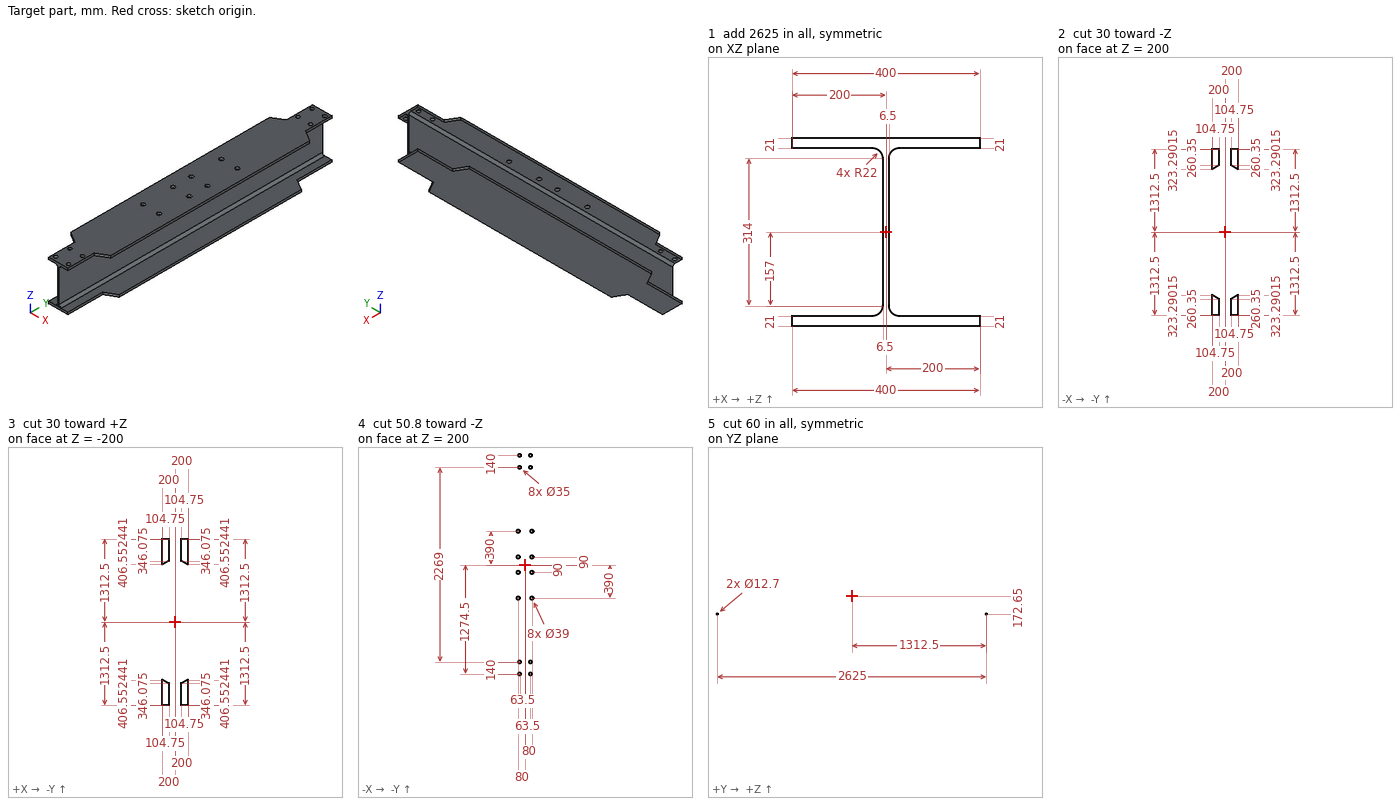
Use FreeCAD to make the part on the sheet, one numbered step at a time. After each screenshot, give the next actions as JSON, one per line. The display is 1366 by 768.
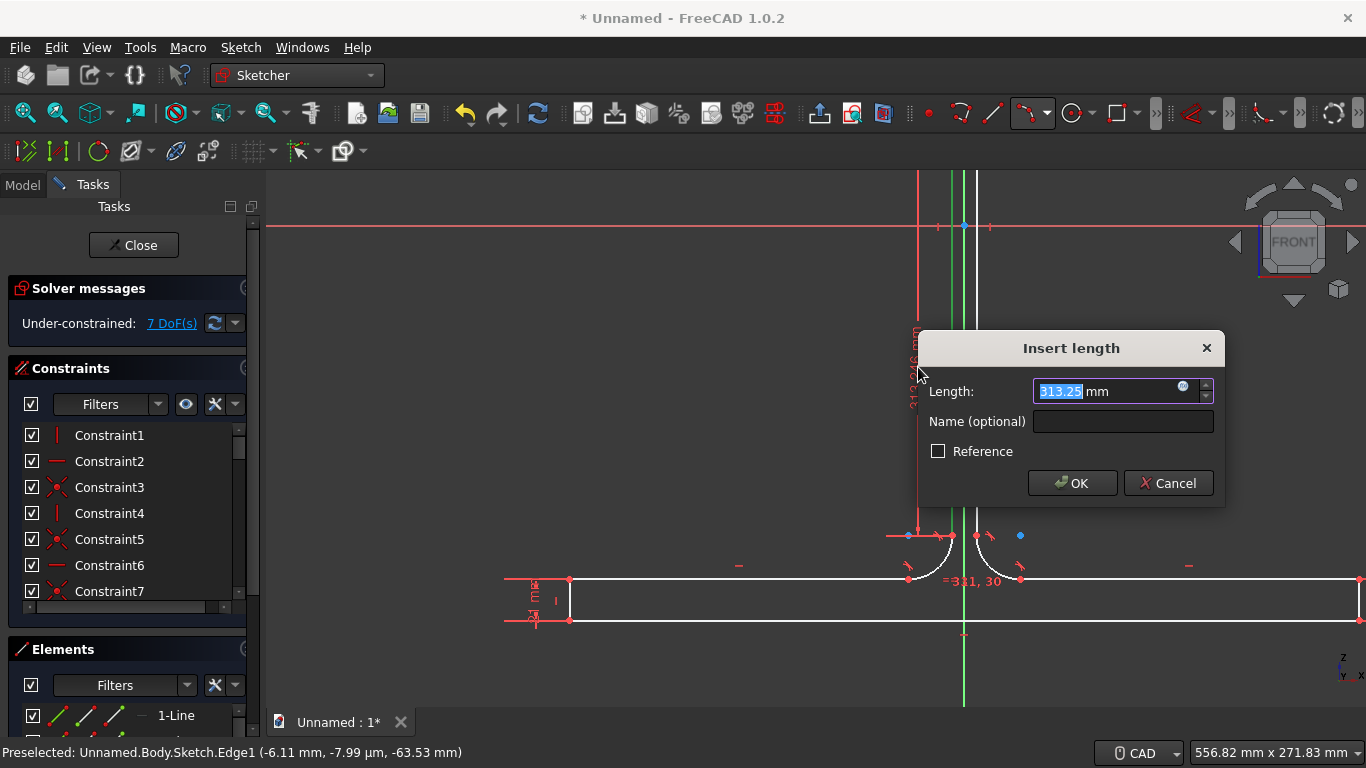
{"action": "type", "text": "314"}
{"action": "key", "text": "Return"}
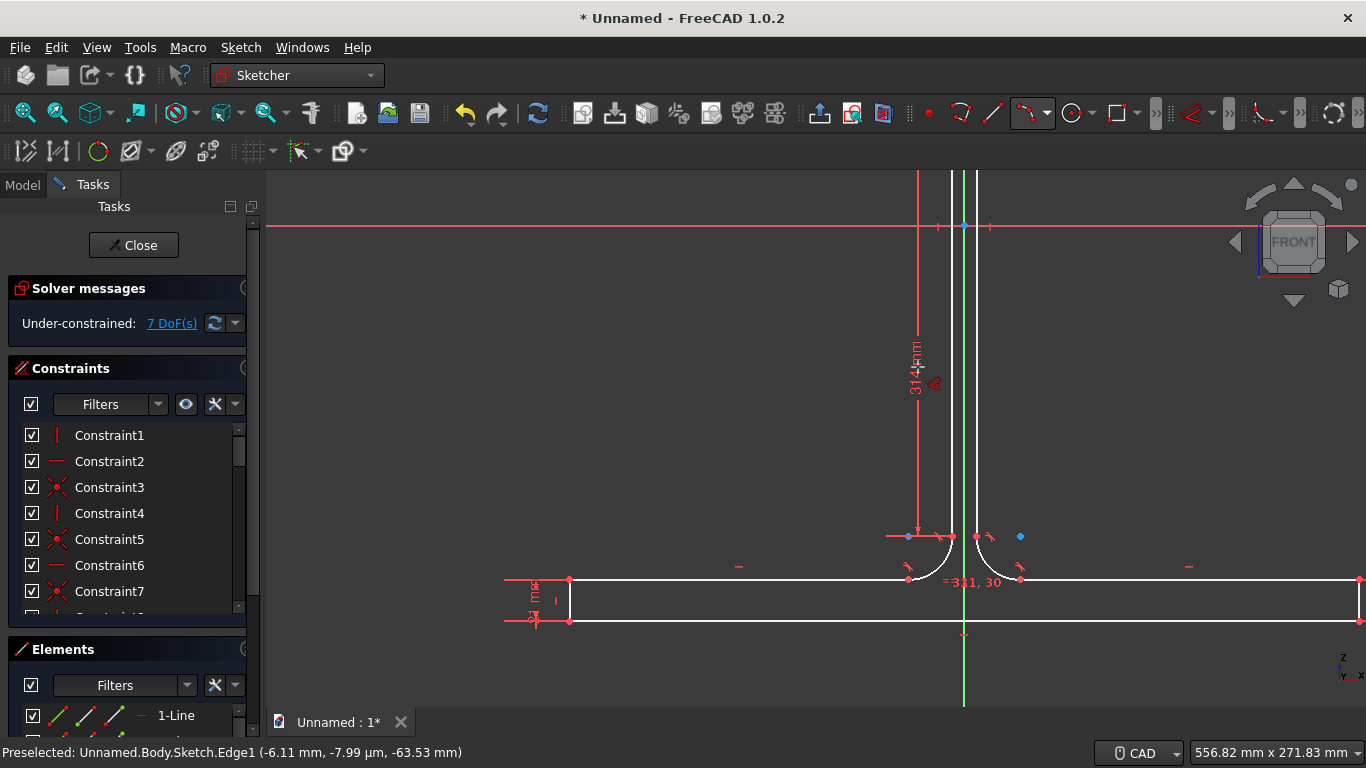
{"action": "scroll", "coordinate": [571, 612], "scroll_direction": "down", "scroll_amount": 4}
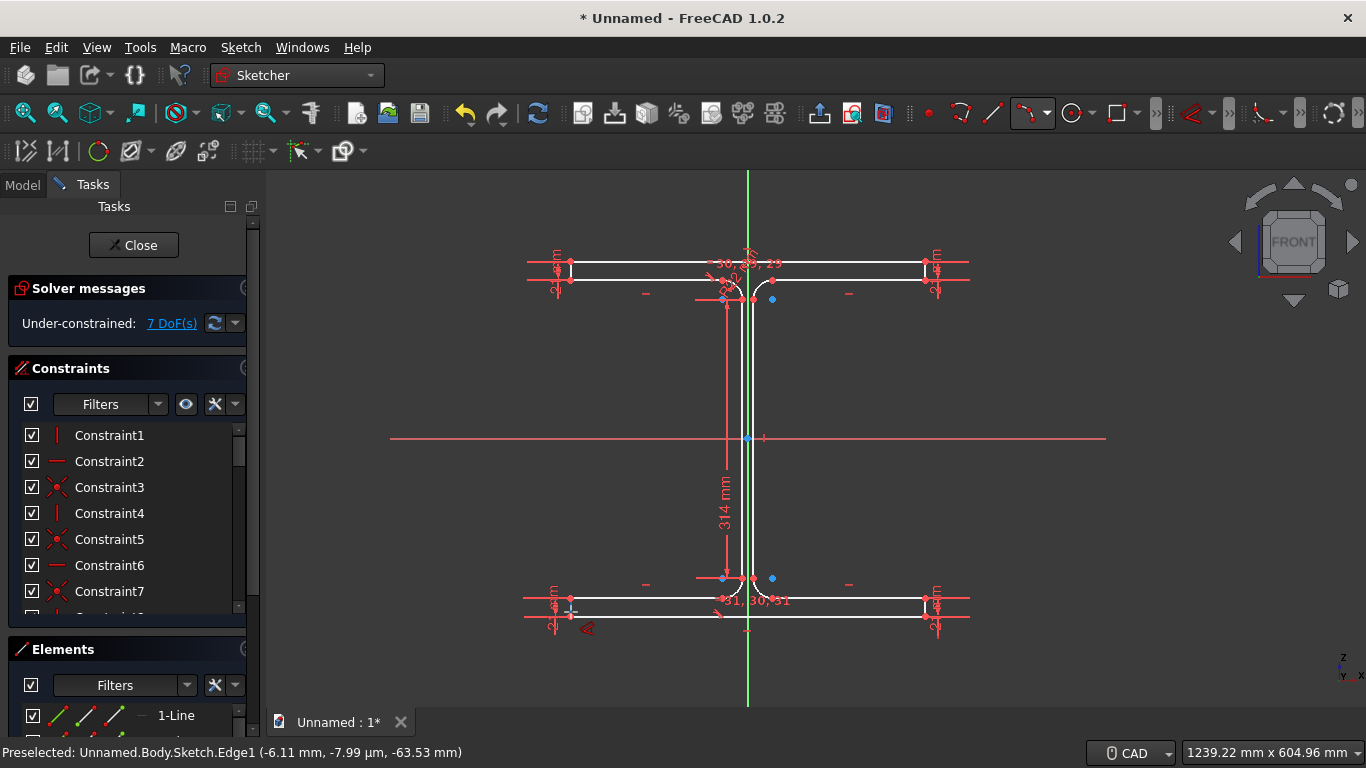
{"action": "left_click", "coordinate": [677, 262]}
{"action": "left_click", "coordinate": [666, 228]}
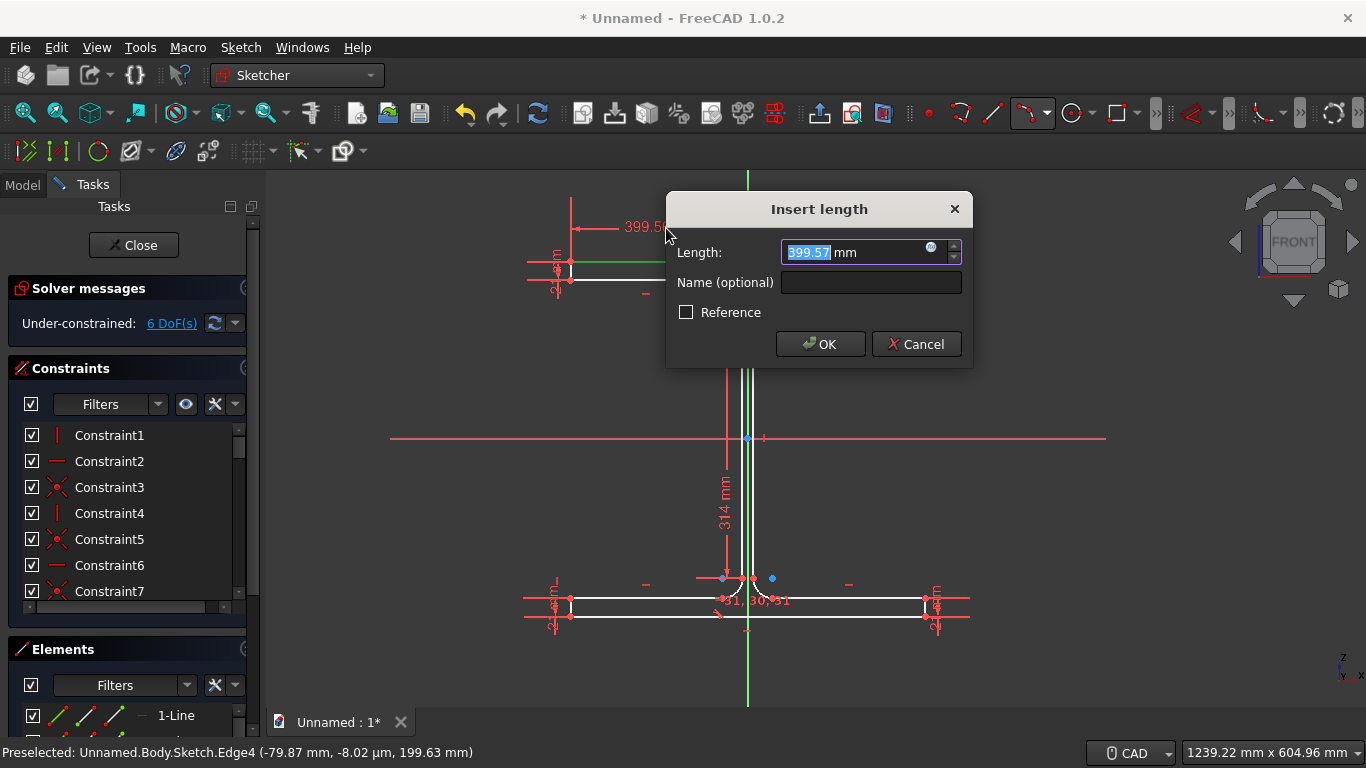
{"action": "type", "text": "400"}
{"action": "key", "text": "Return"}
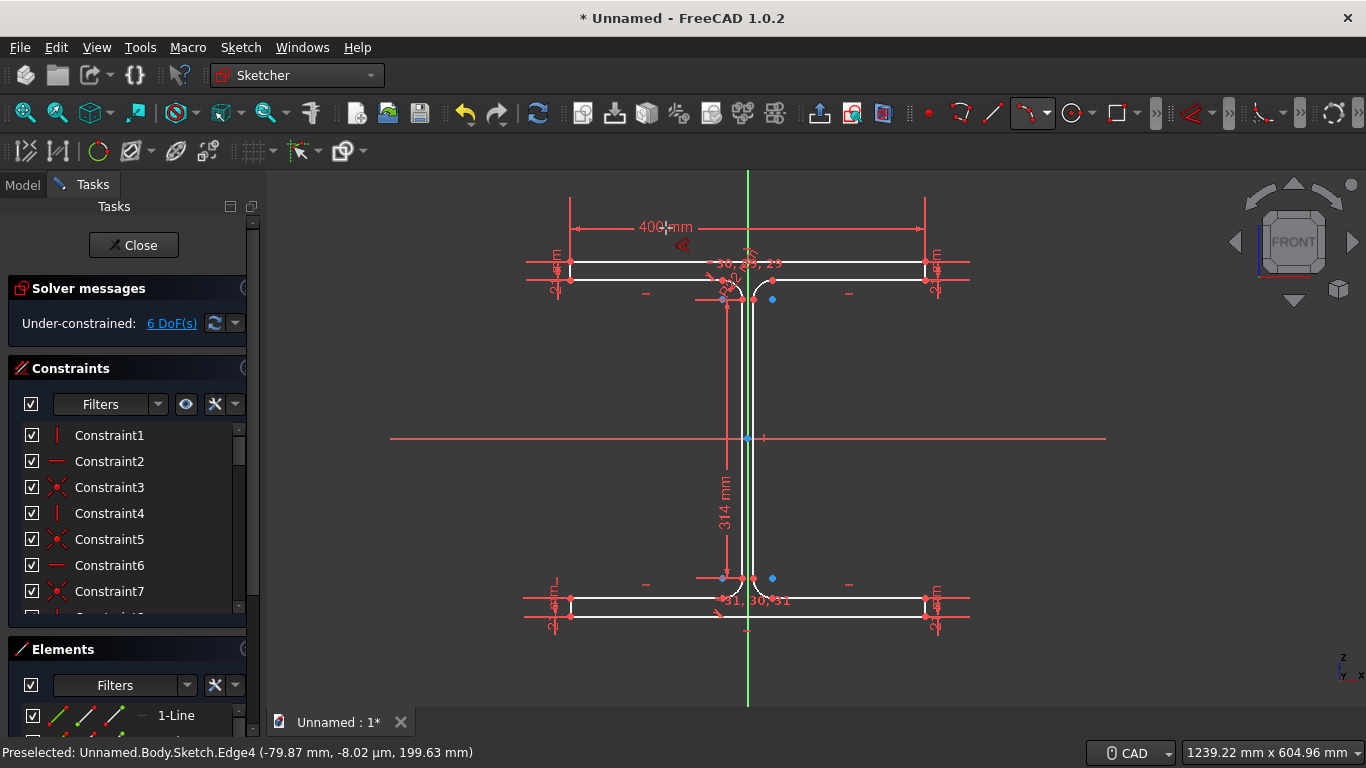
{"action": "left_click", "coordinate": [819, 617]}
{"action": "left_click", "coordinate": [666, 651]}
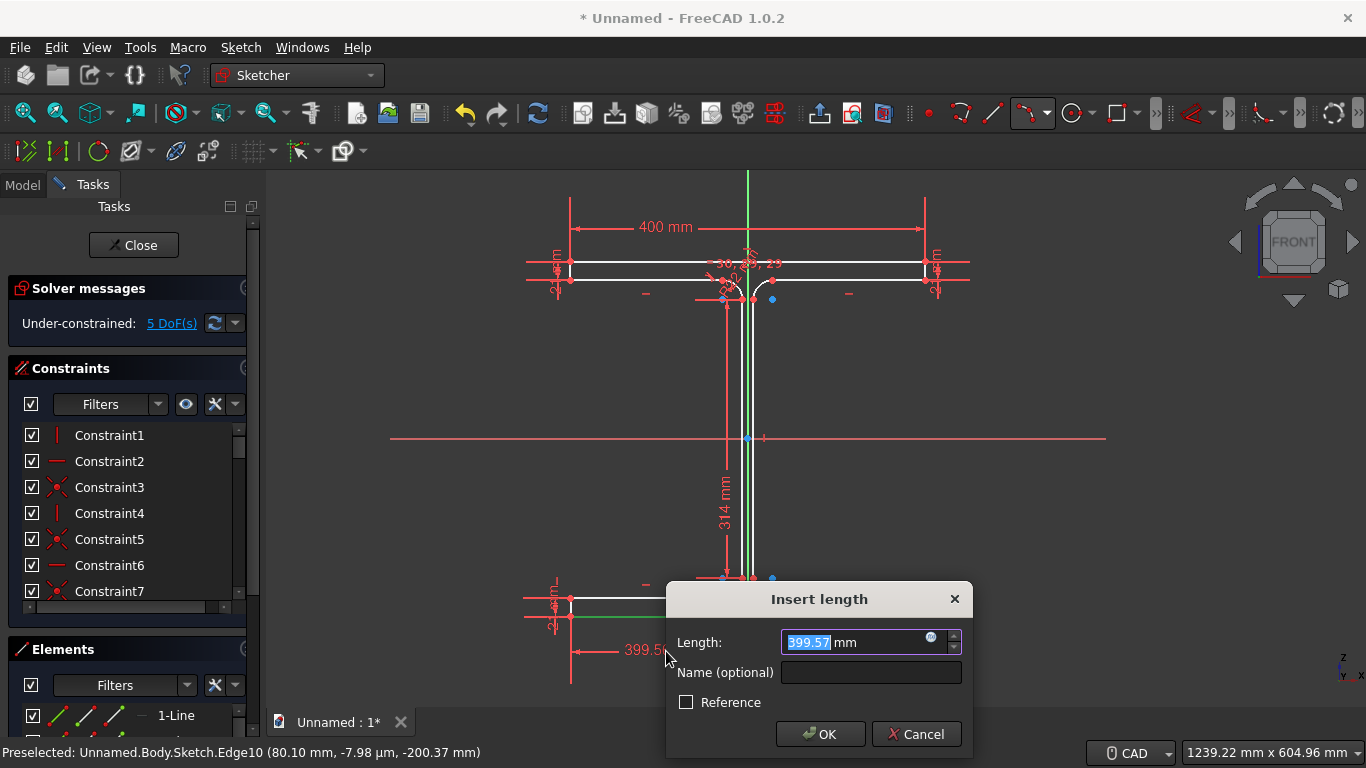
{"action": "type", "text": "400"}
{"action": "key", "text": "Return"}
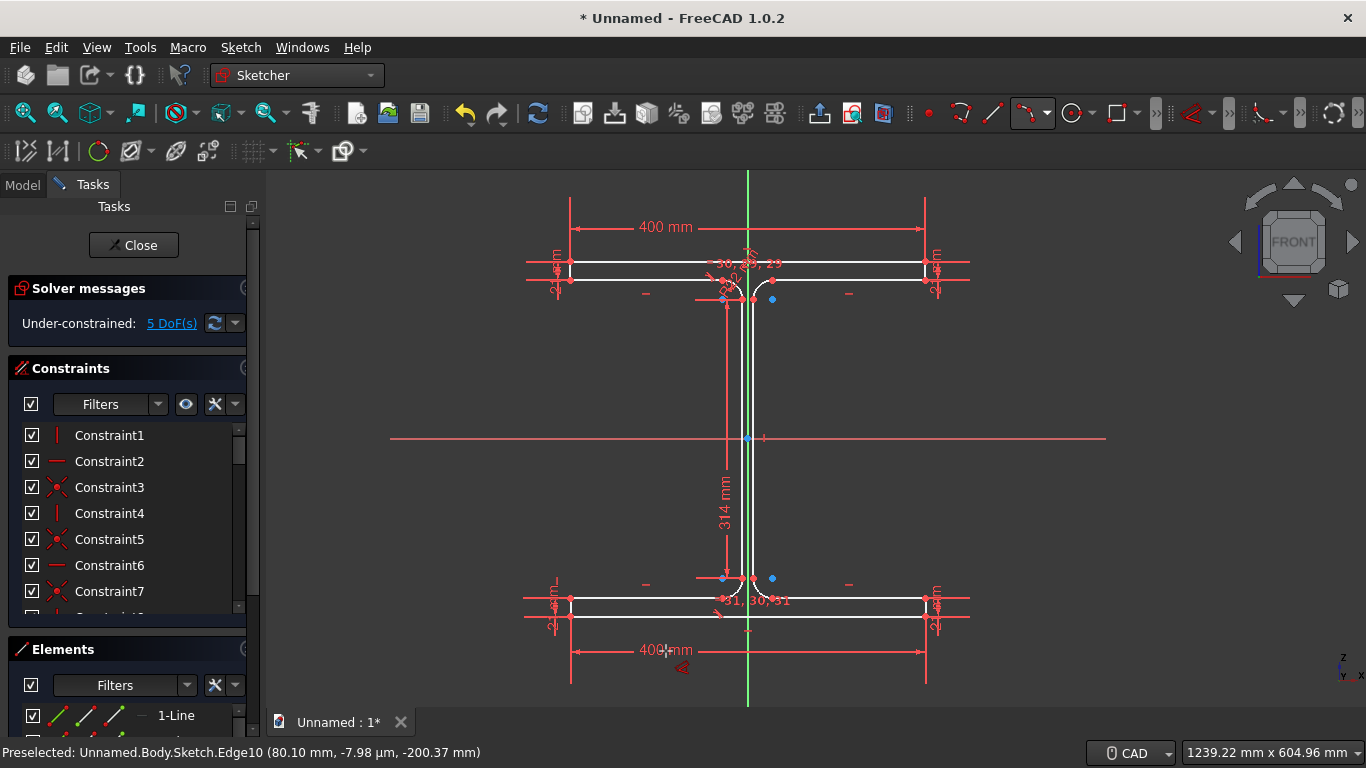
{"action": "scroll", "coordinate": [742, 578], "scroll_direction": "up", "scroll_amount": 10}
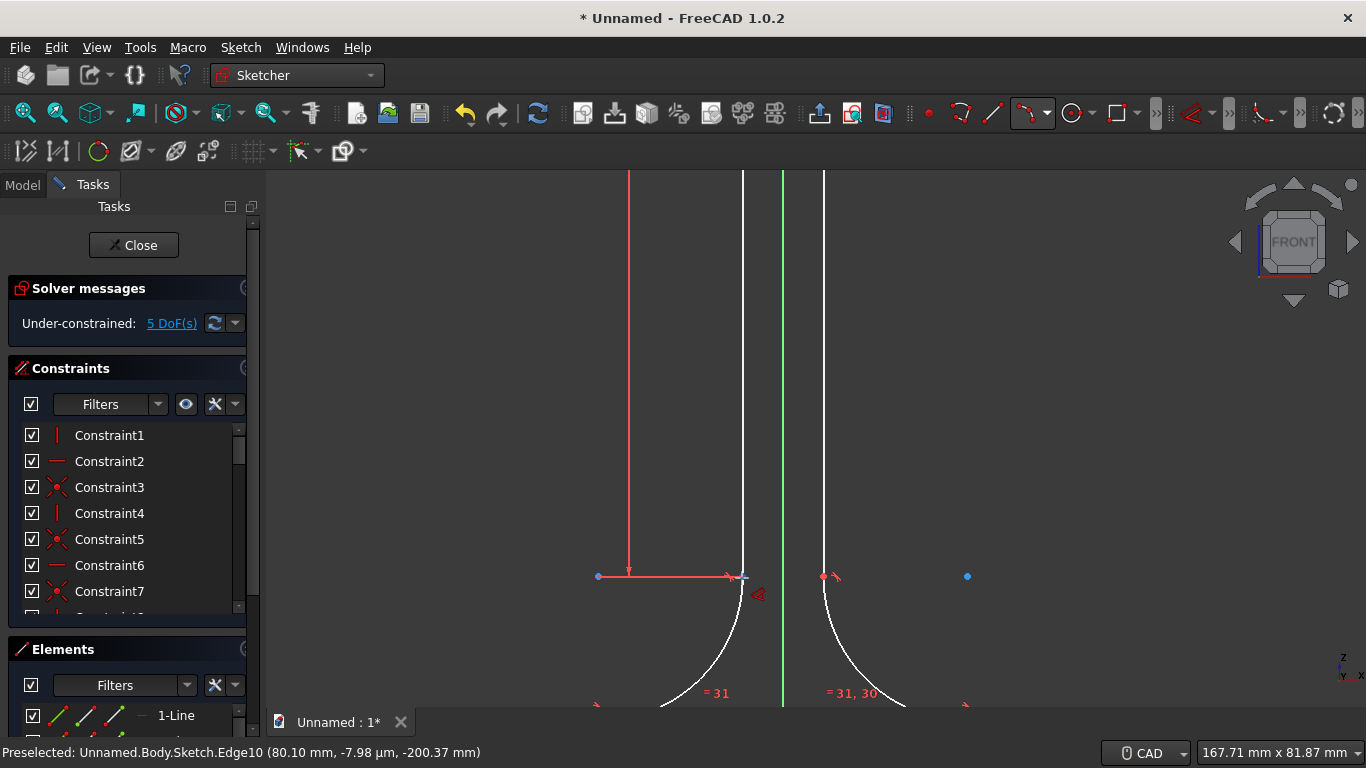
{"action": "left_click", "coordinate": [743, 577]}
{"action": "left_click", "coordinate": [763, 611]}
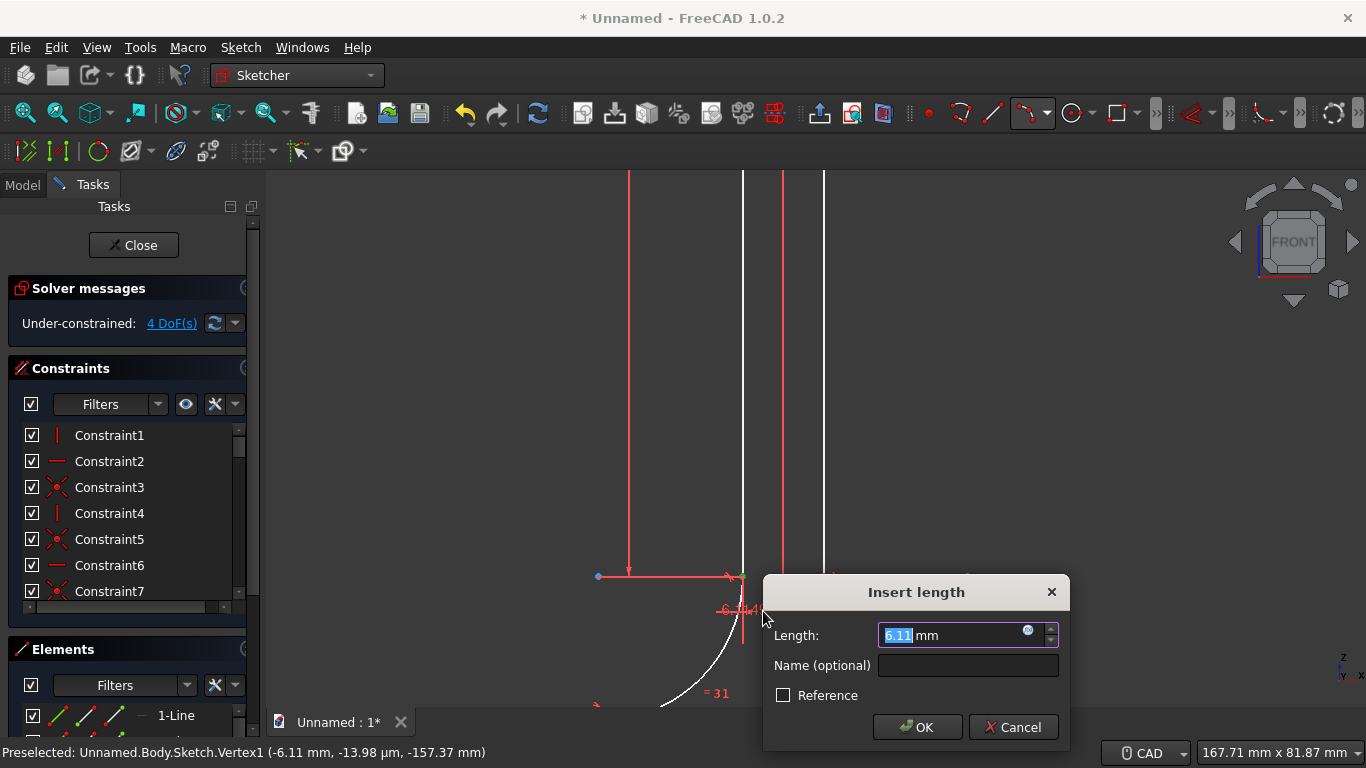
{"action": "type", "text": "6.5"}
{"action": "key", "text": "Return"}